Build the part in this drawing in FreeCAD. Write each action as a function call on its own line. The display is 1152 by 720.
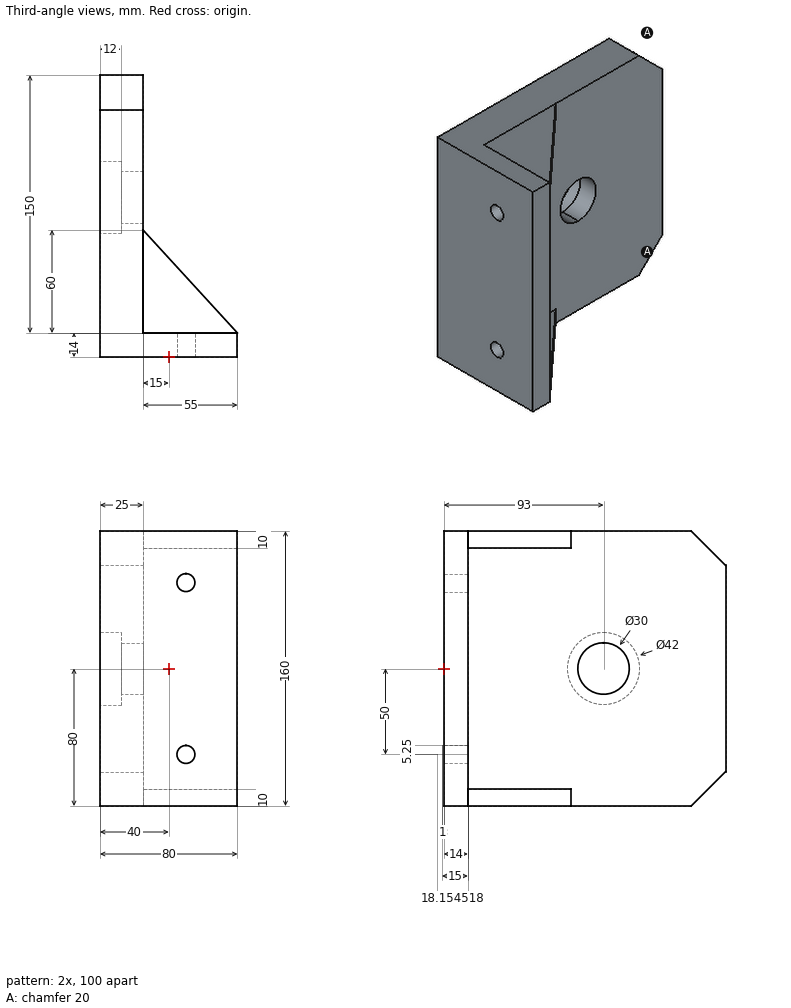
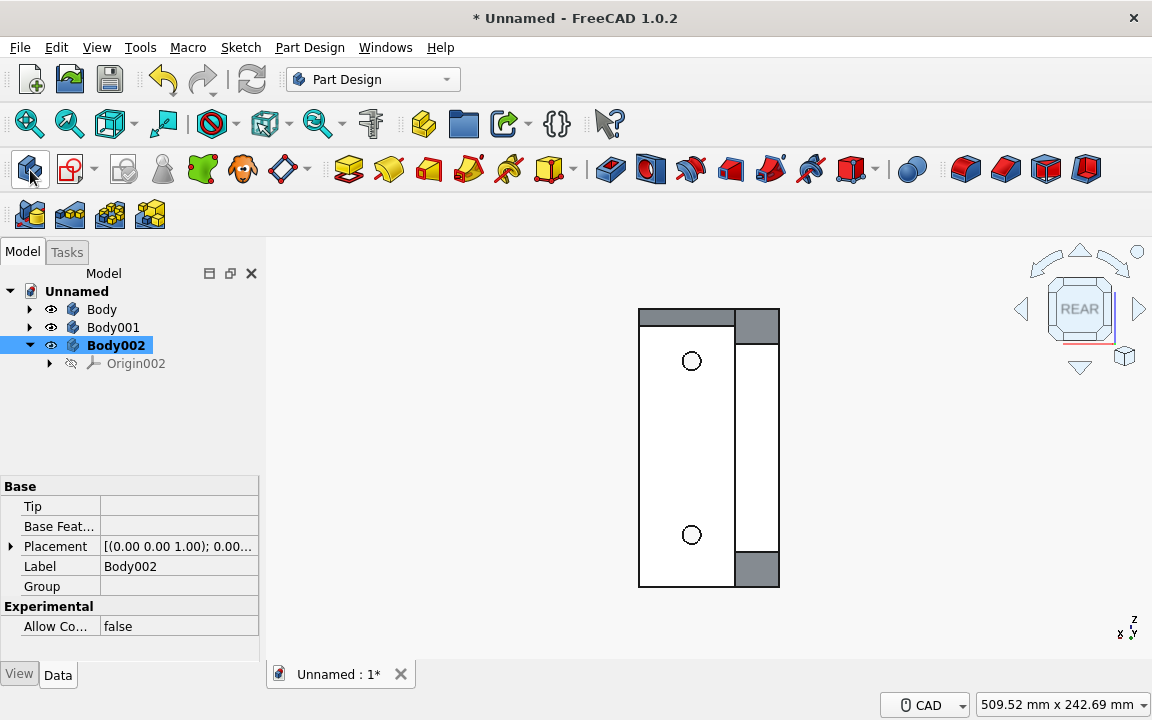
click(50, 363)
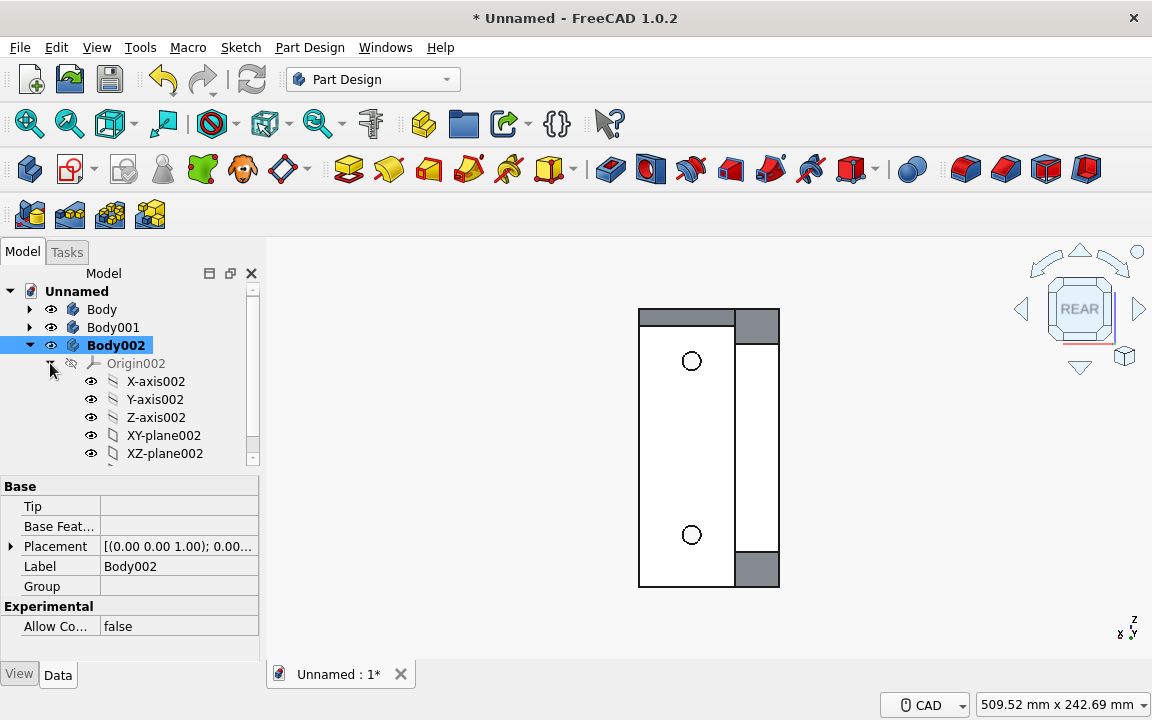
click(136, 435)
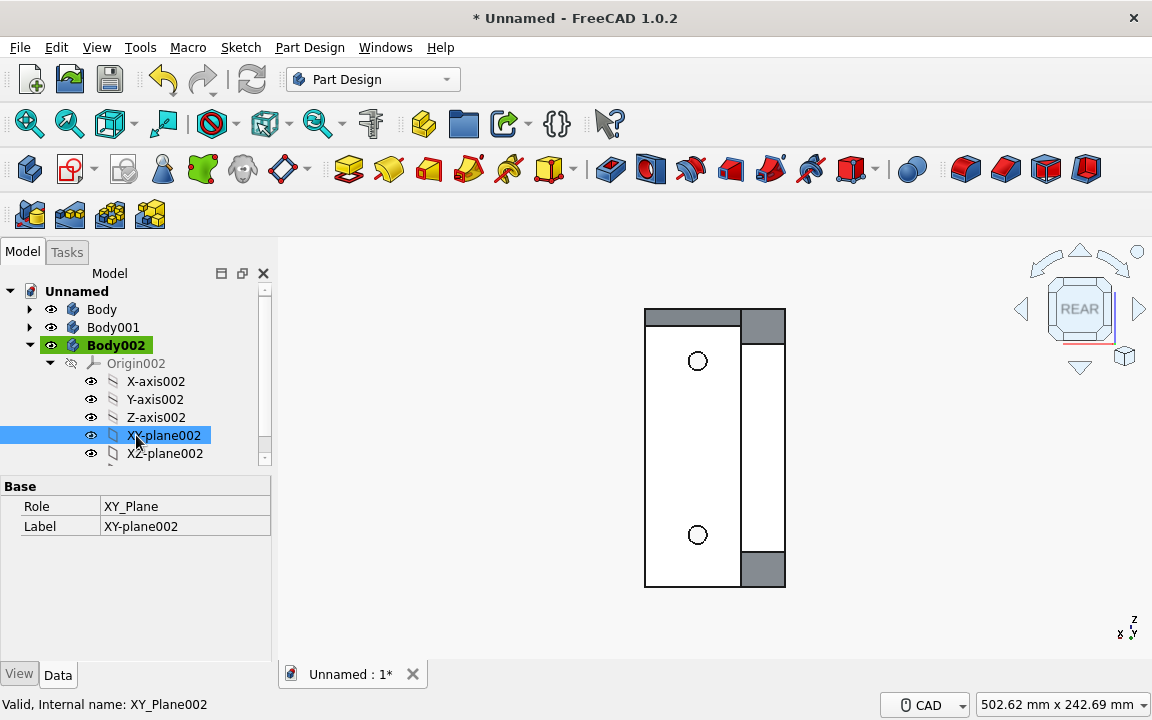
click(284, 170)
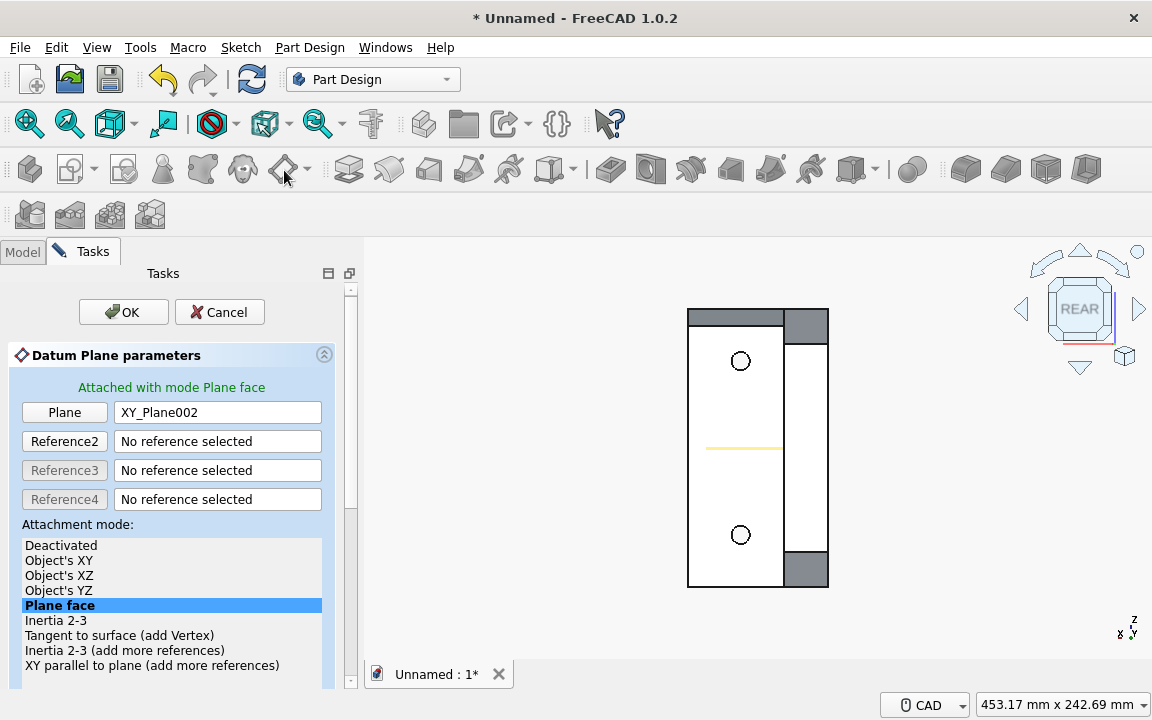
scroll(351, 486, down, 4)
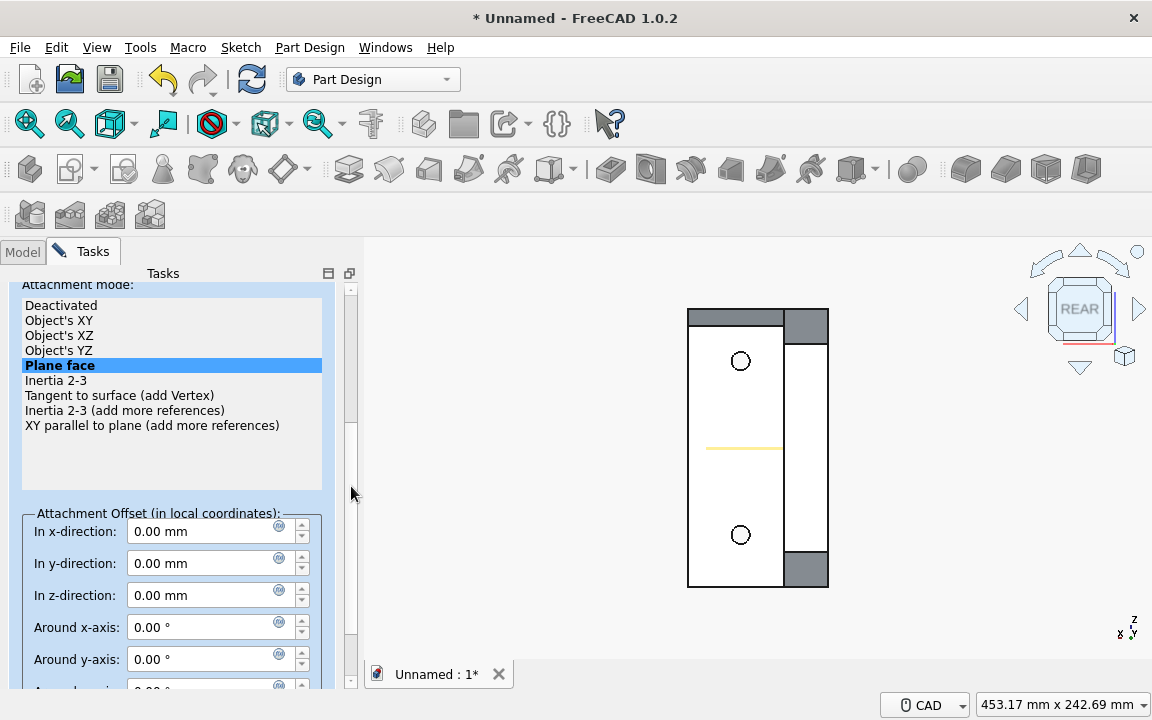
triple_click(210, 595)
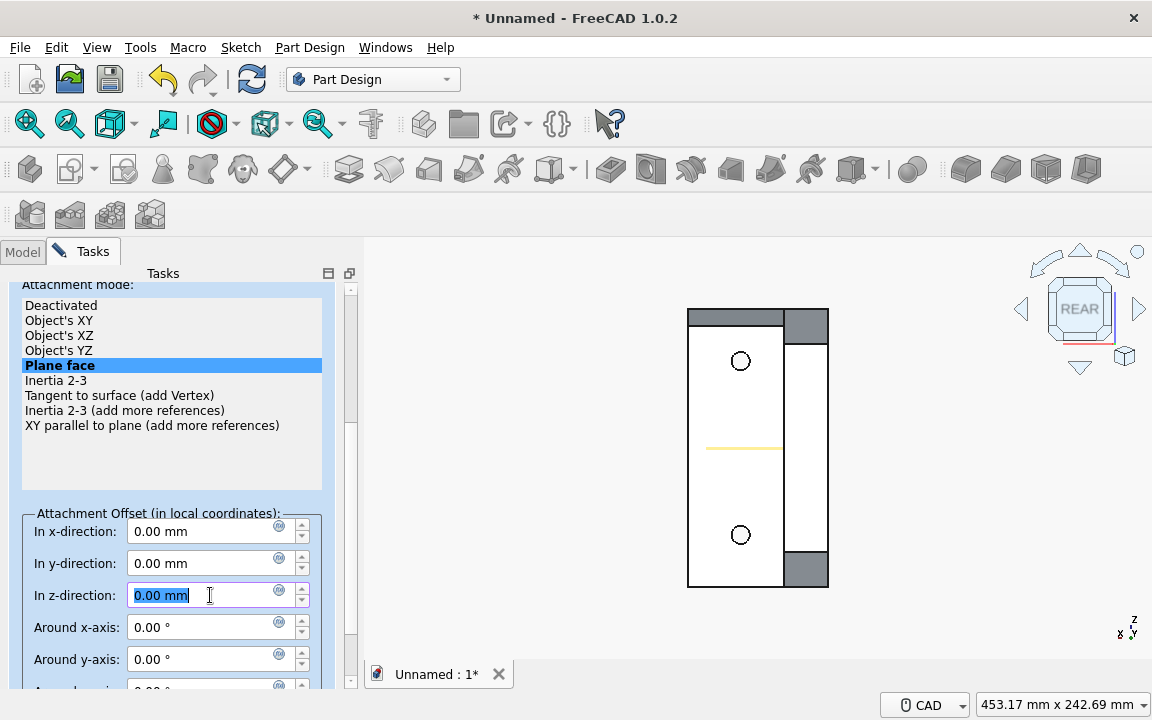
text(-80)
key(Tab)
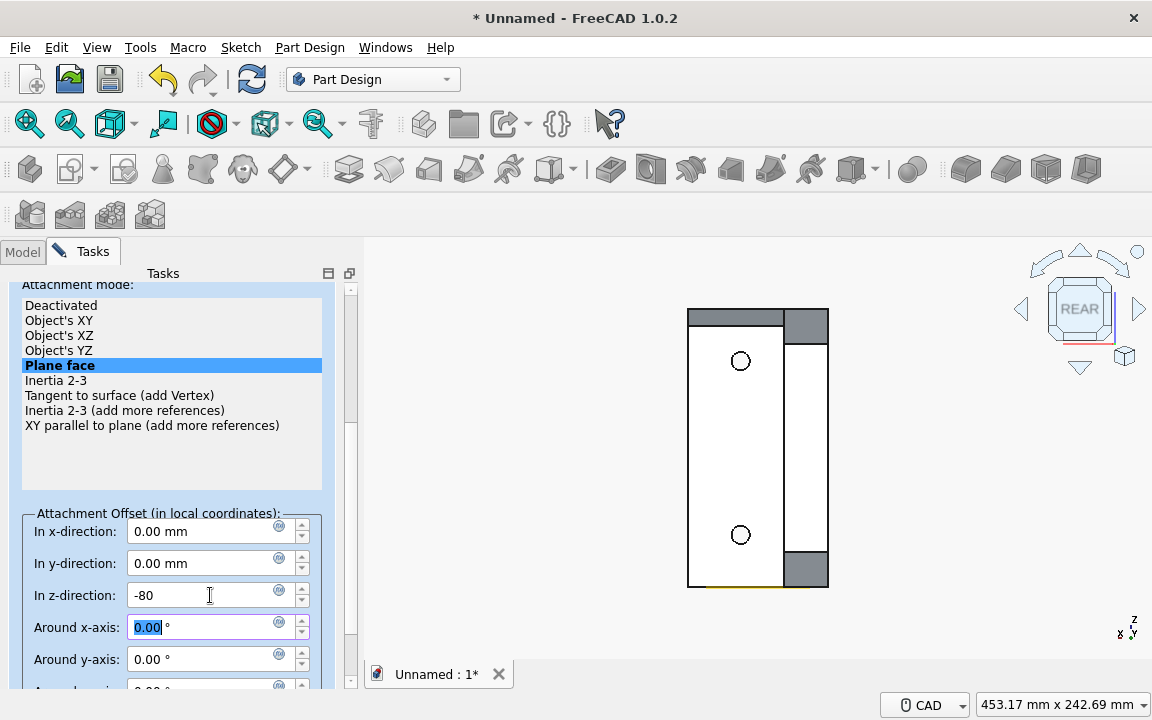
scroll(351, 486, up, 5)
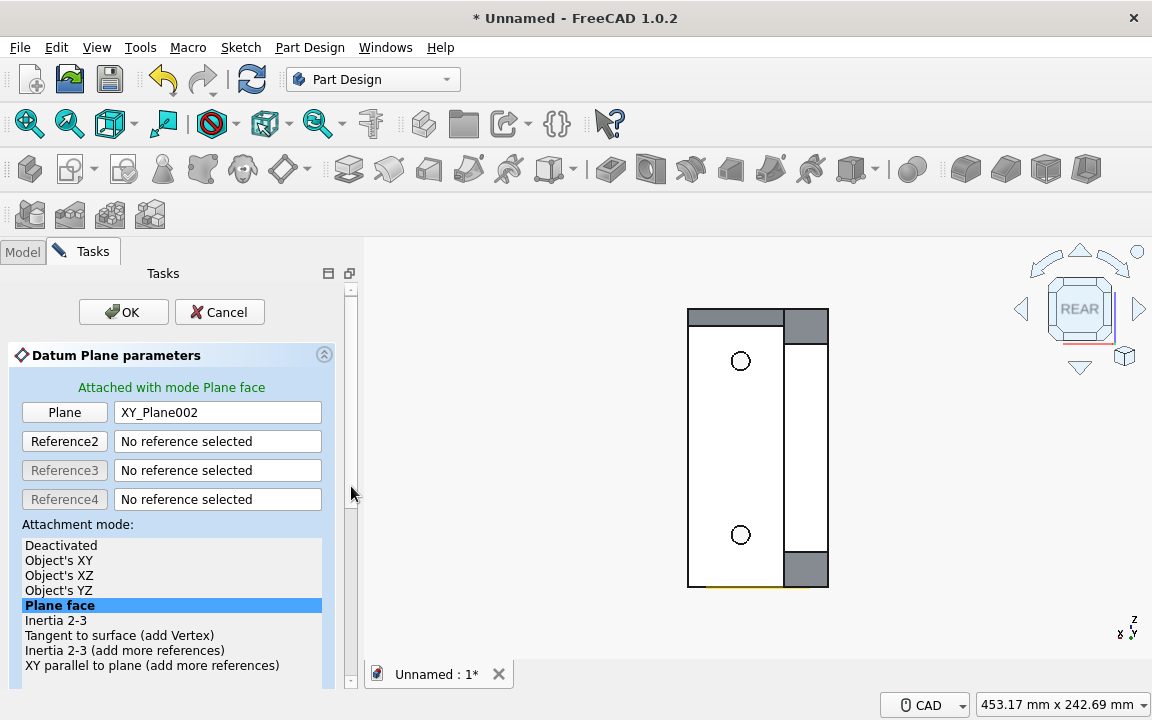
click(124, 312)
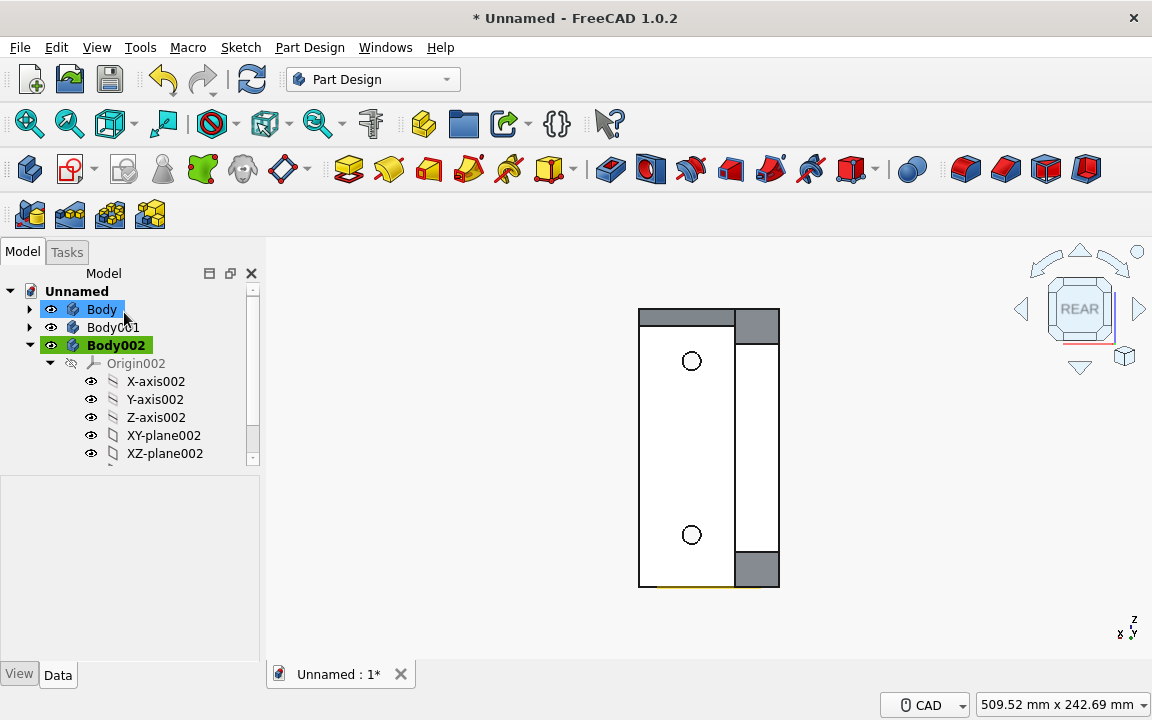
scroll(100, 377, down, 3)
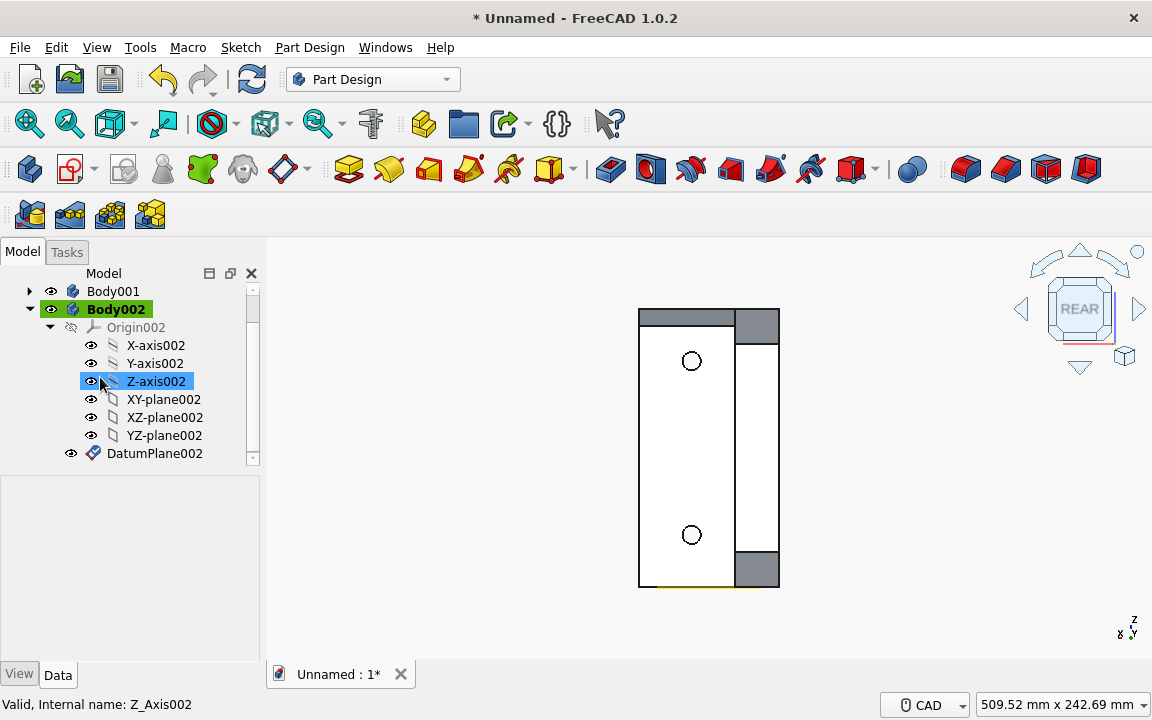
click(116, 453)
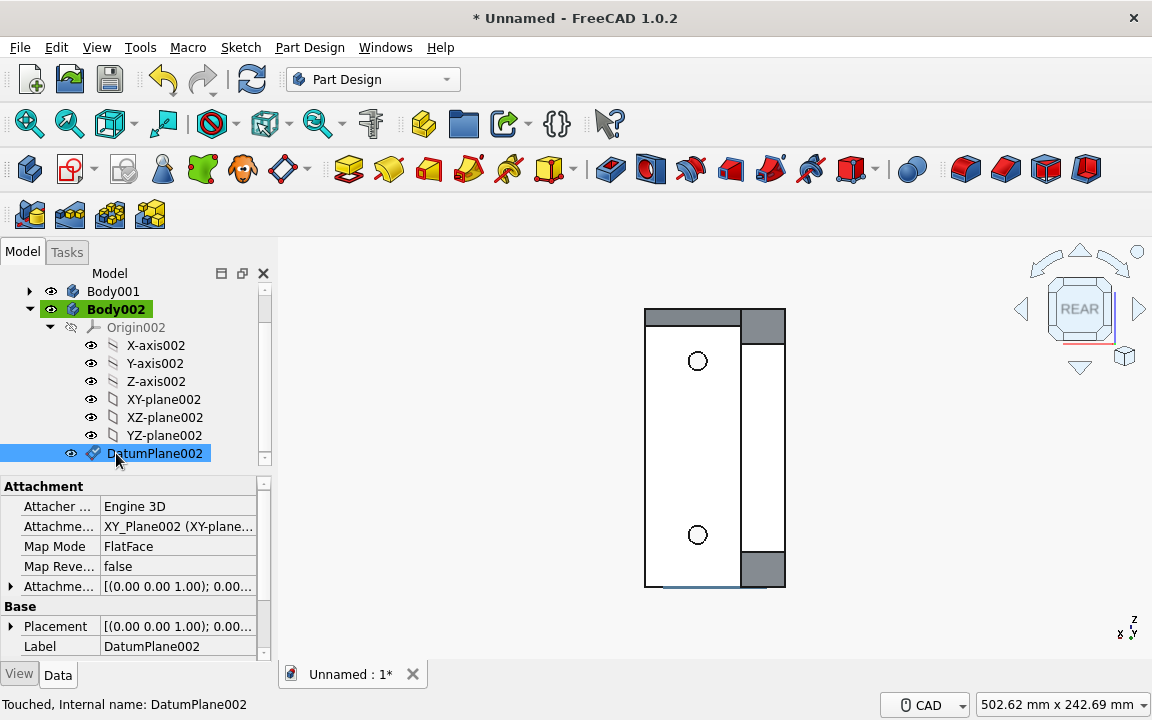
click(70, 170)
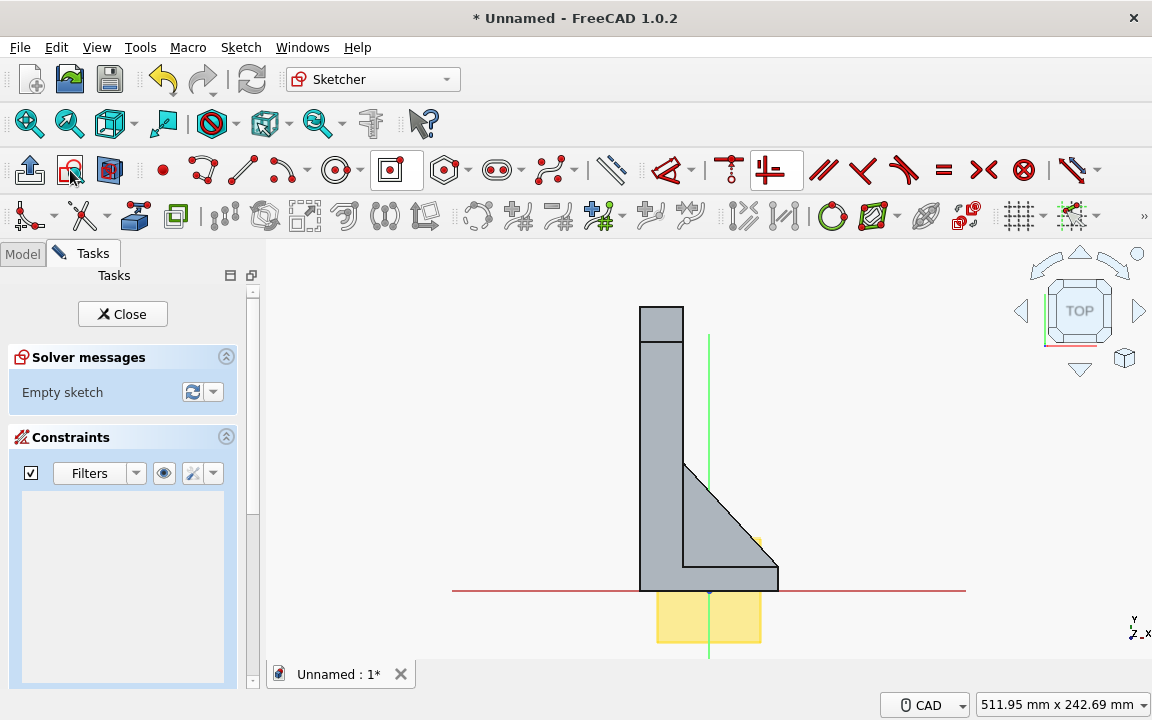
scroll(840, 622, up, 3)